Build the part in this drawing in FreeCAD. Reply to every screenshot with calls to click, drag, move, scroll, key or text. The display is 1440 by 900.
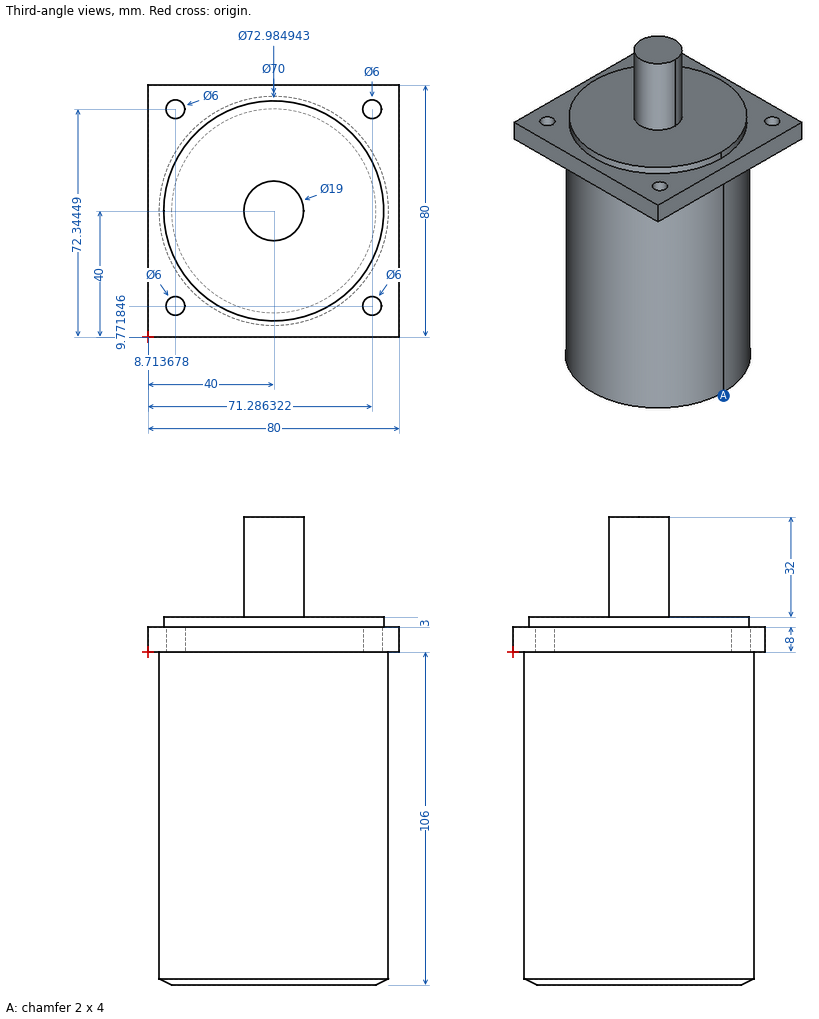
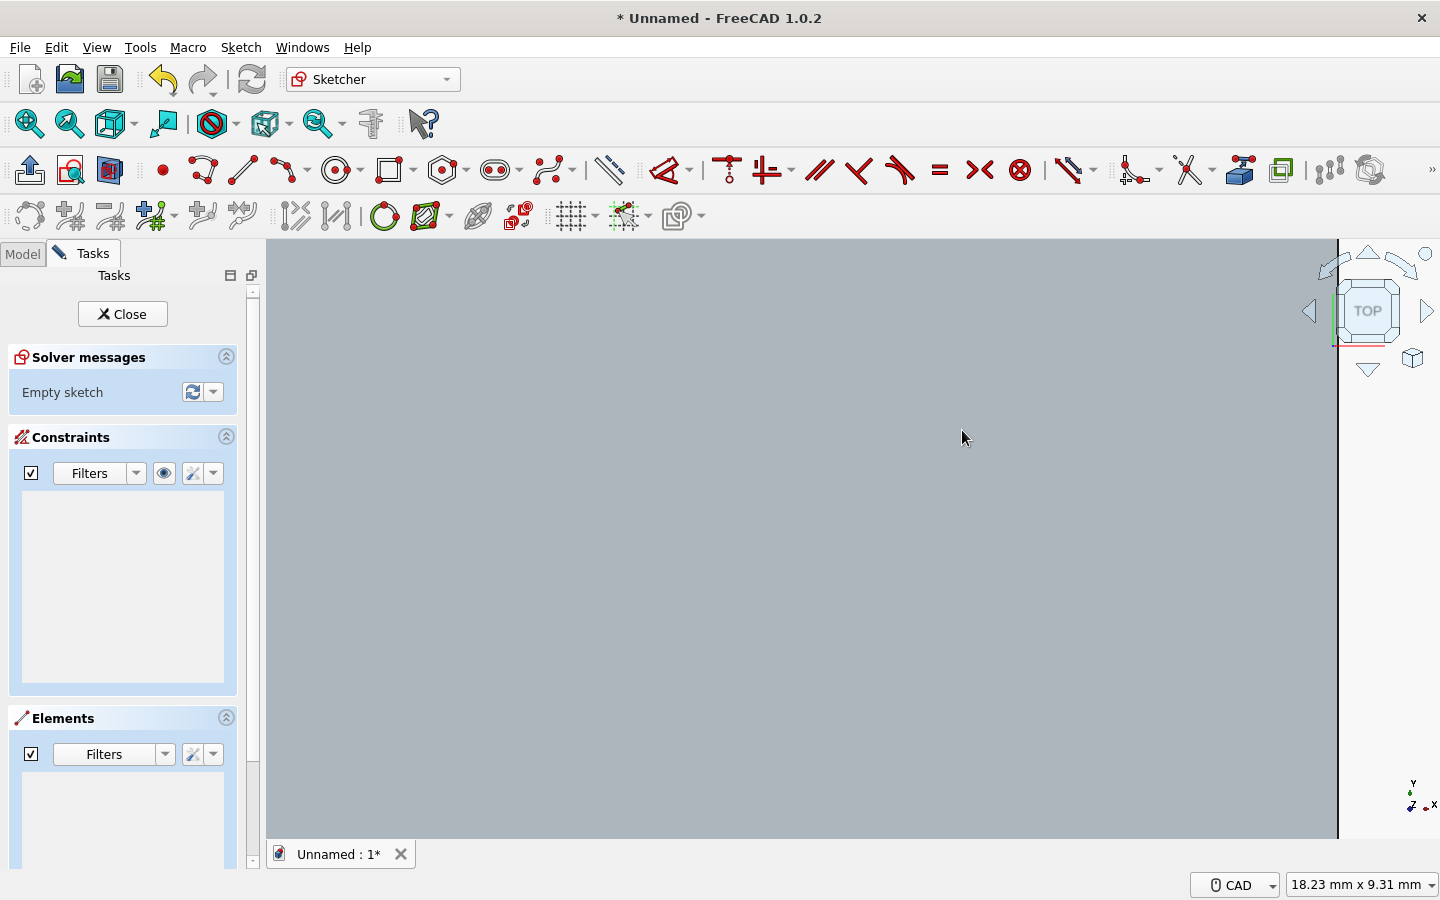
click(336, 170)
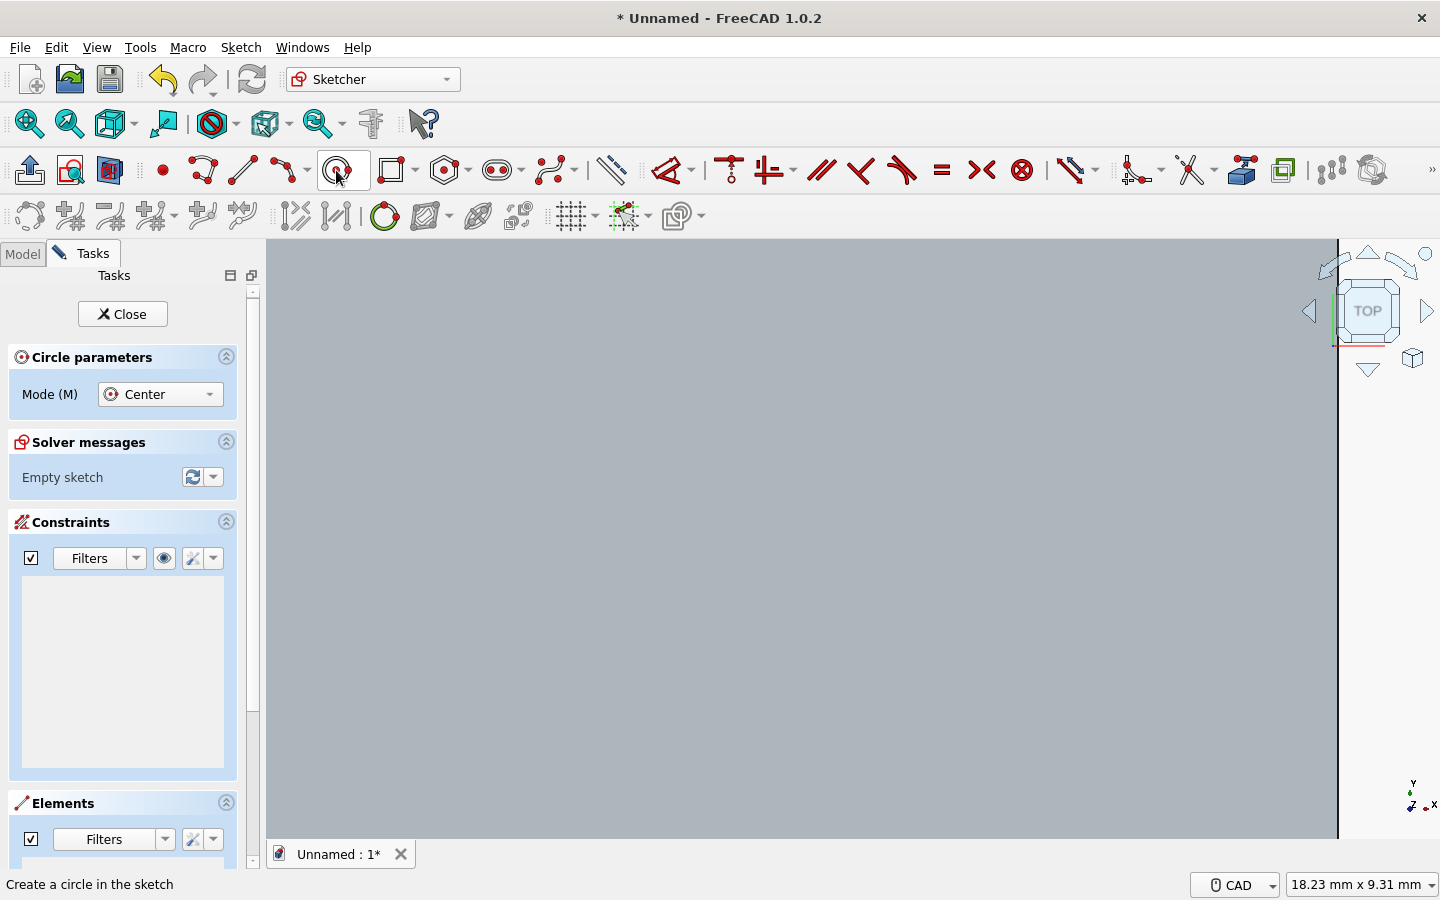
click(777, 530)
move(913, 393)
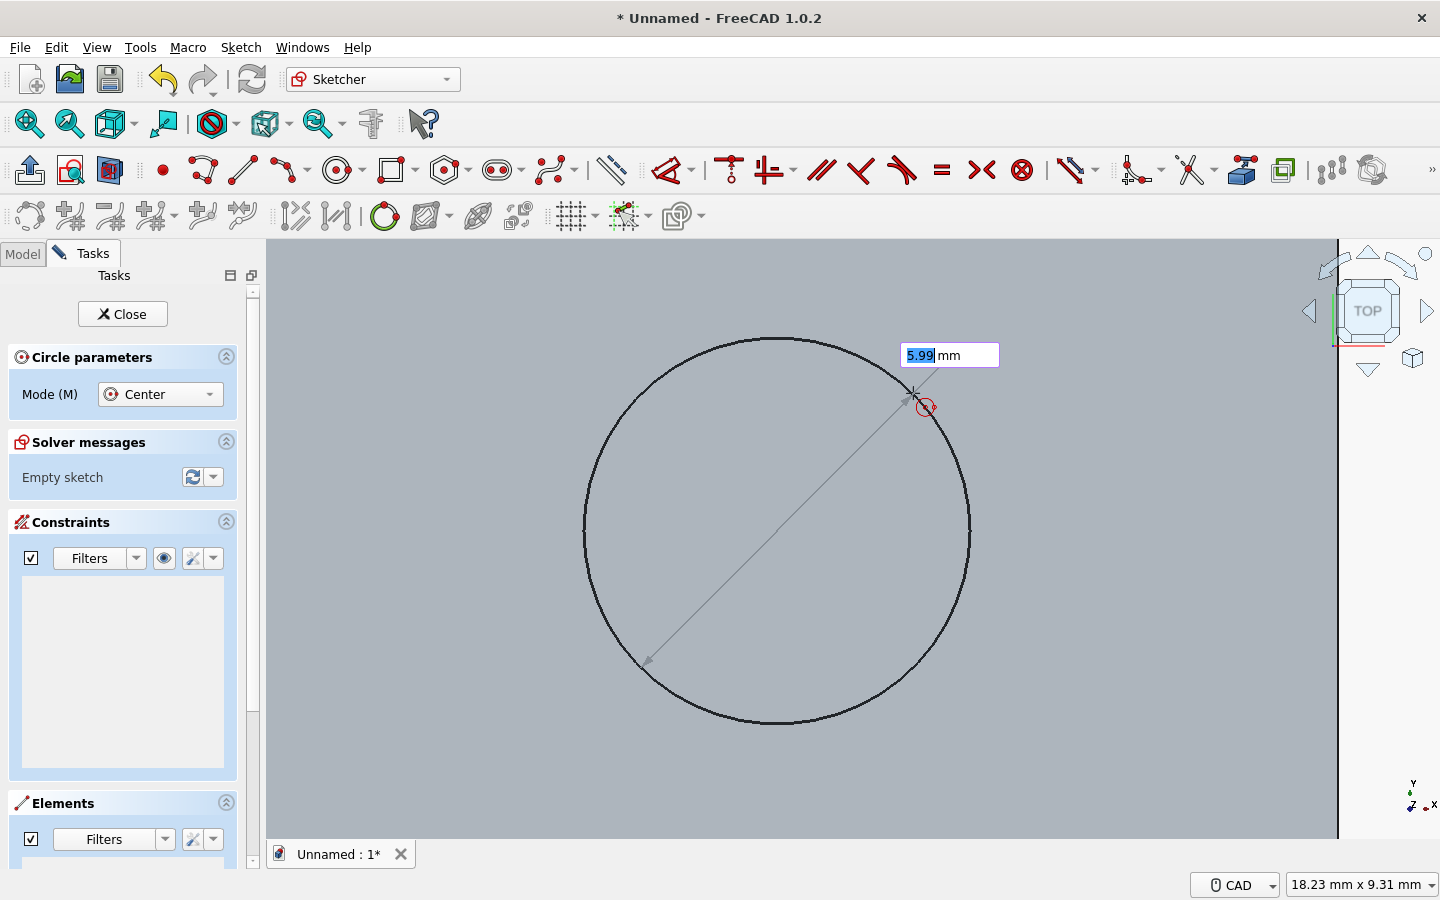
text(6)
key(Return)
key(Escape)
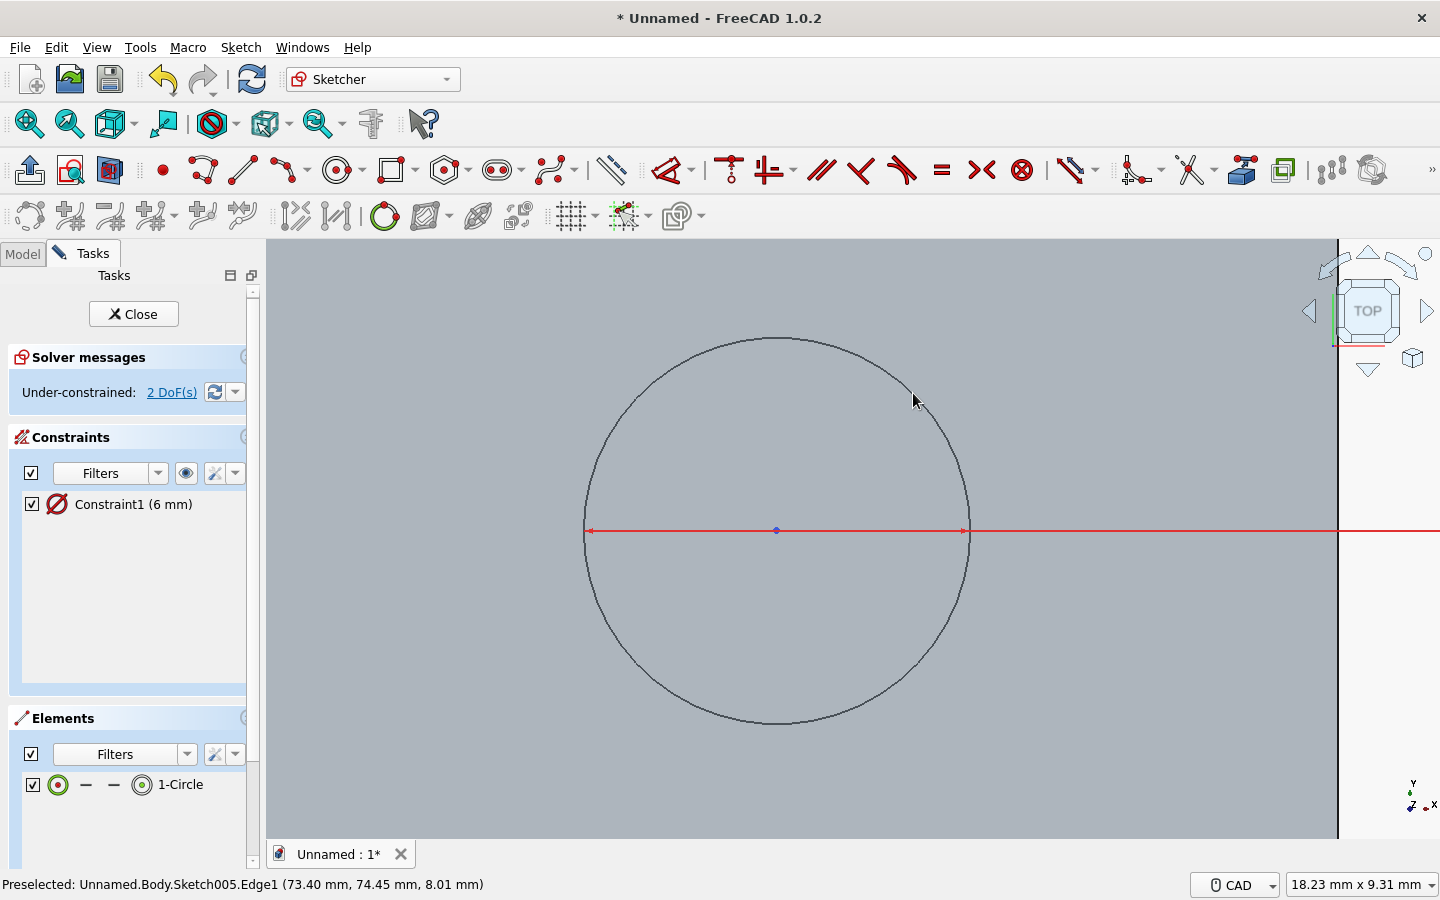
click(666, 170)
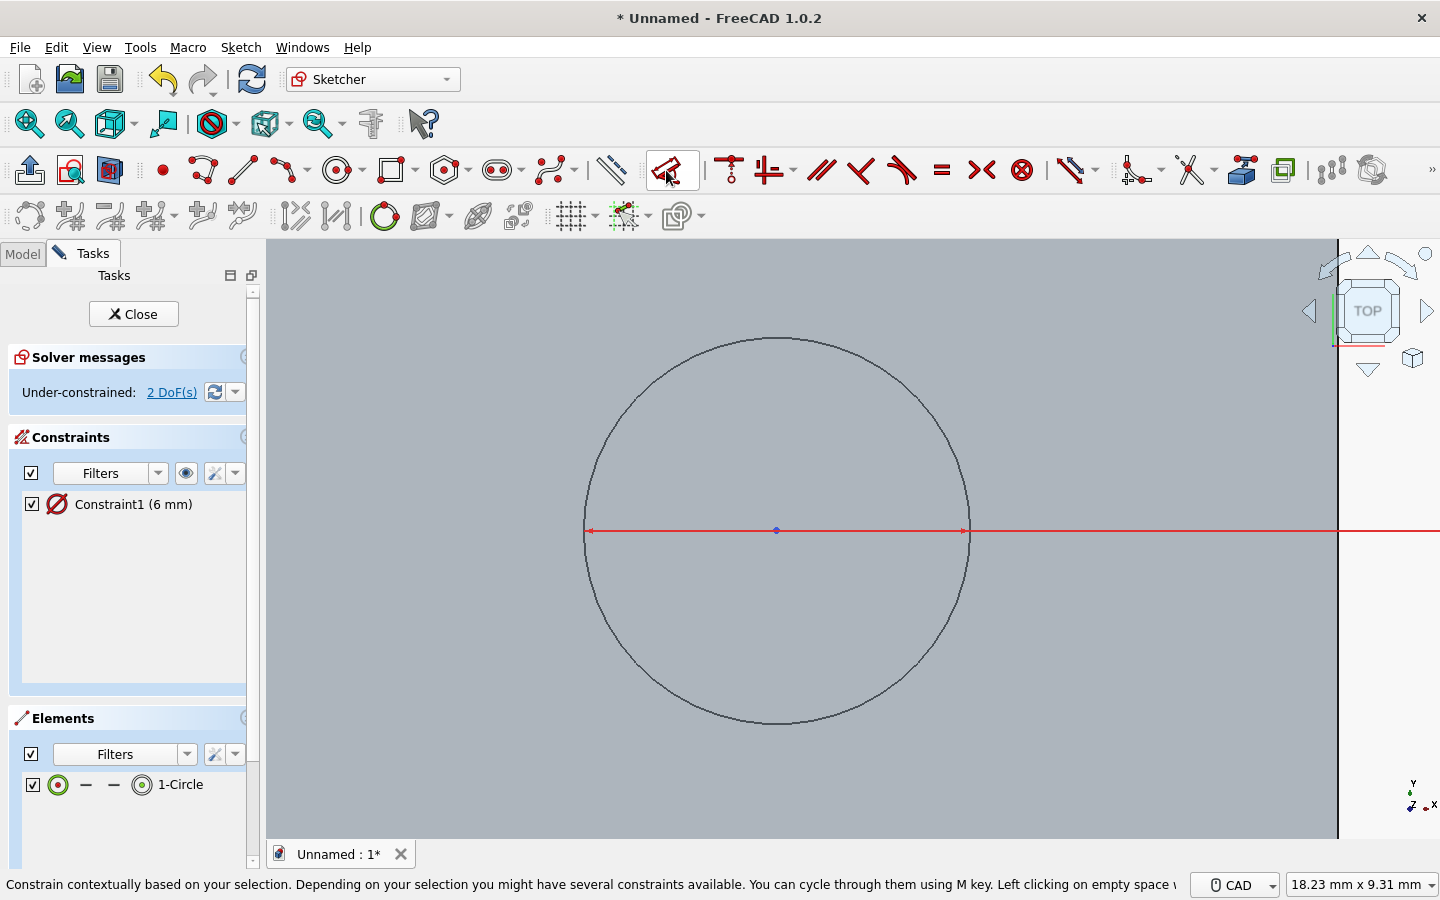
click(777, 531)
click(811, 671)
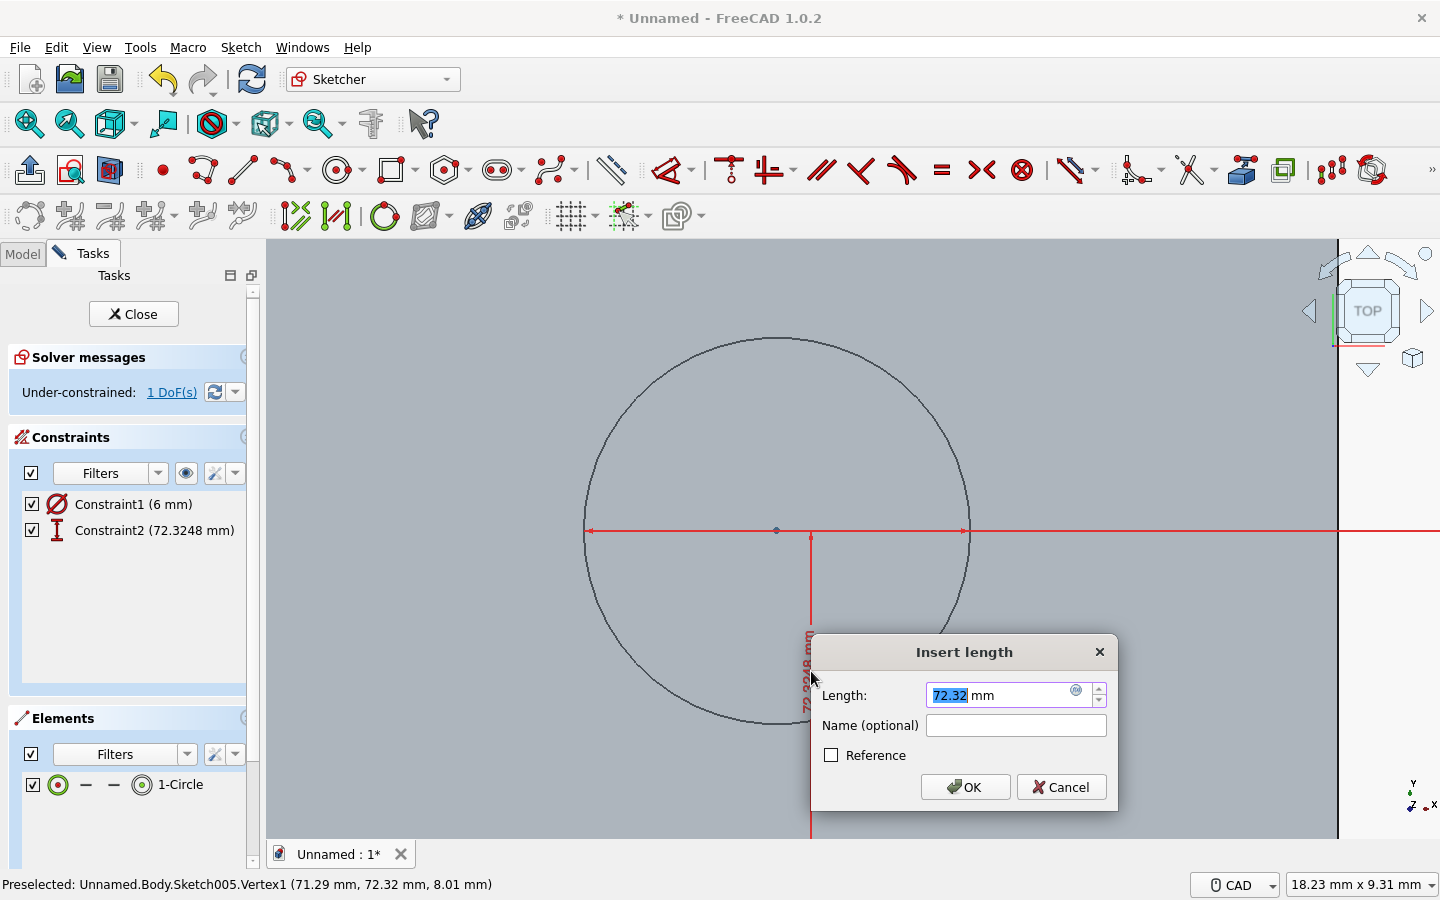
text(72.34449)
key(Return)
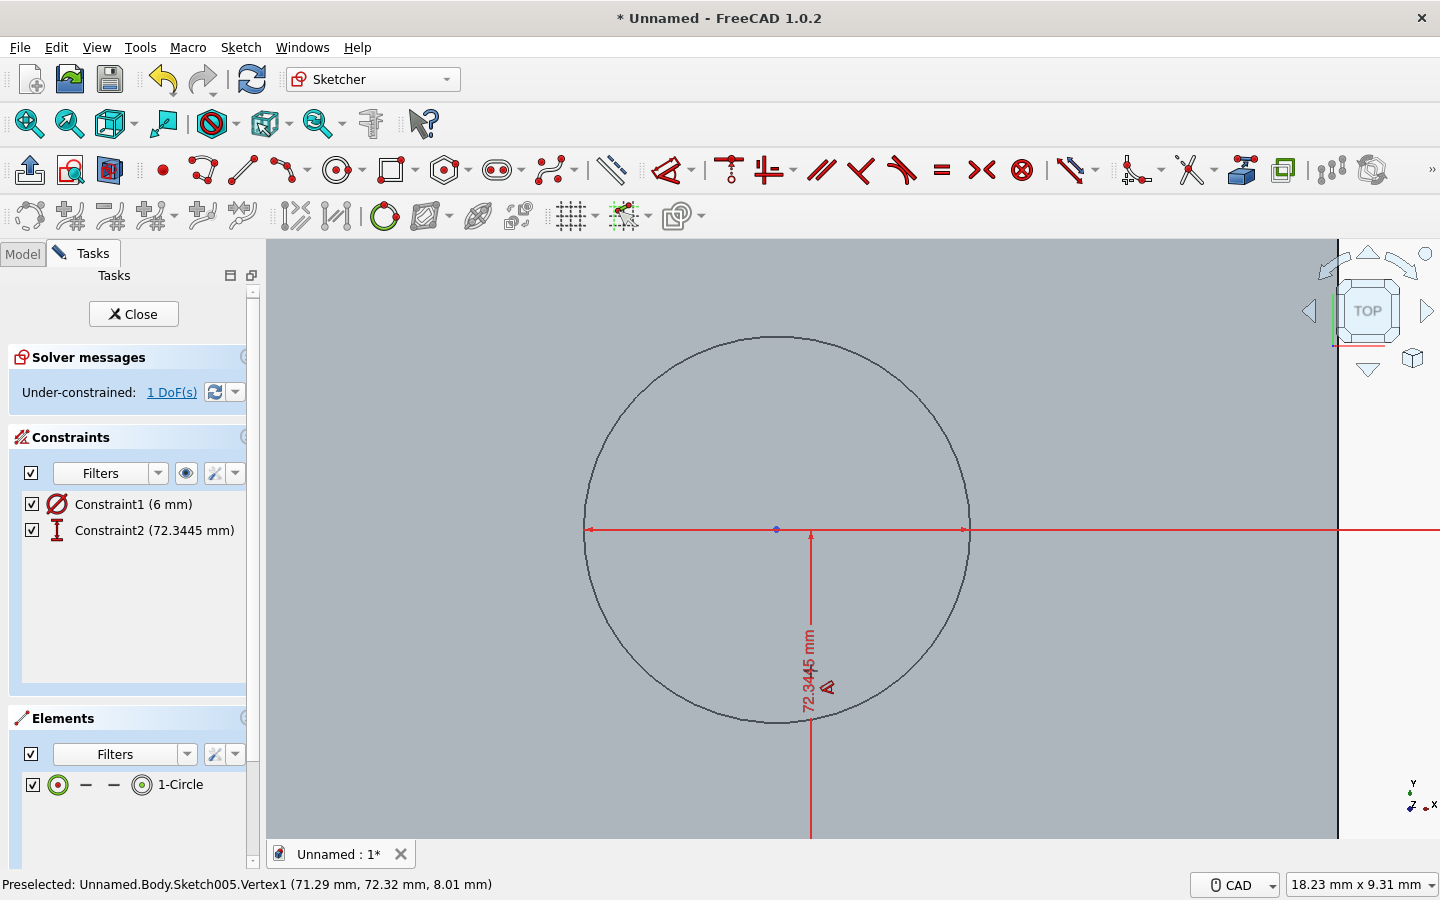
click(777, 530)
click(535, 496)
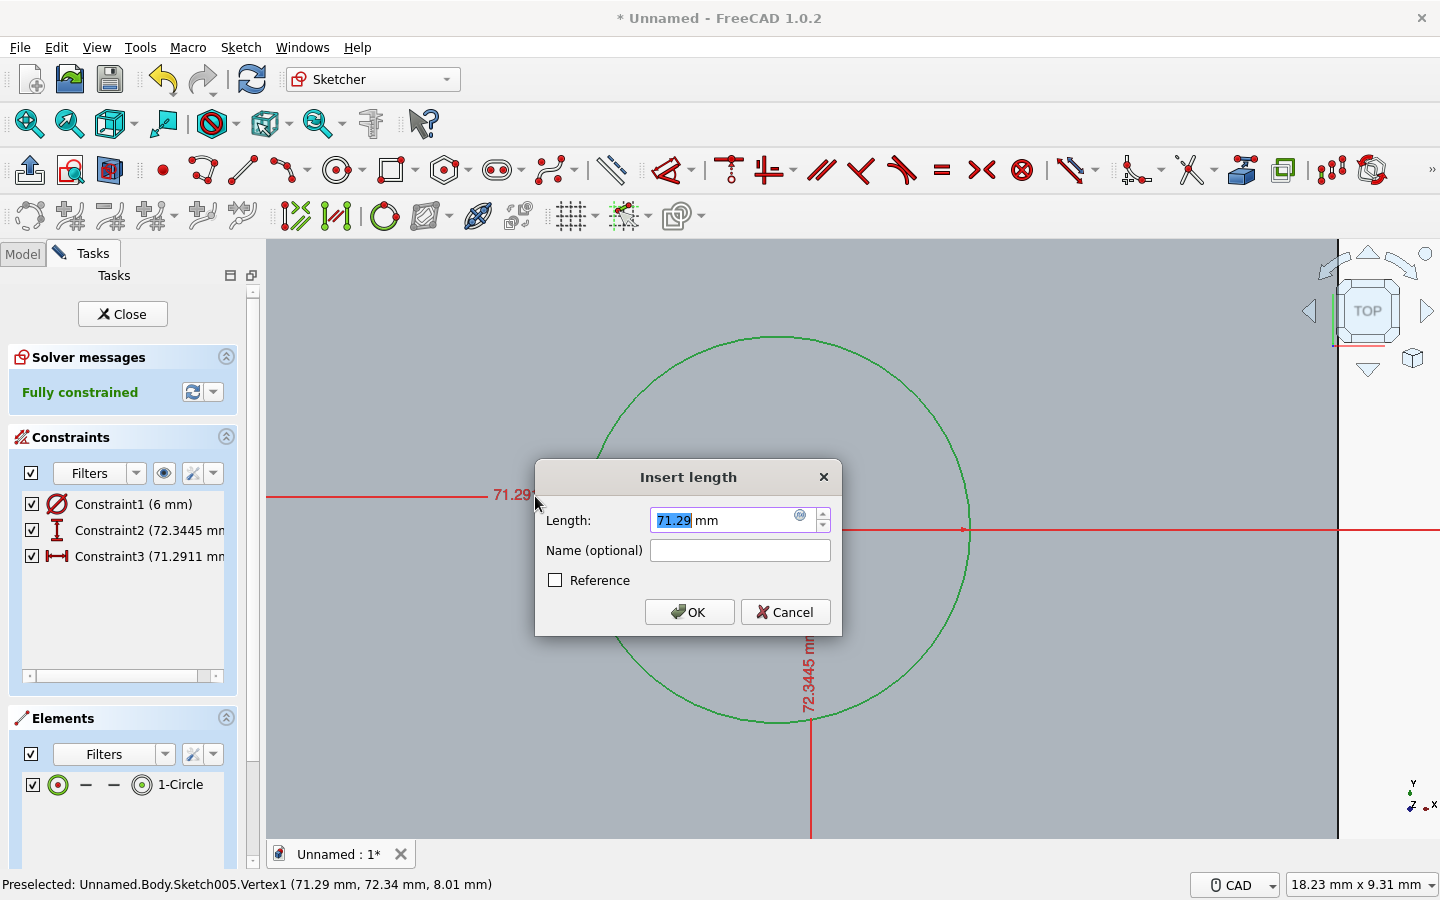
text(71.286322)
key(Return)
key(Escape)